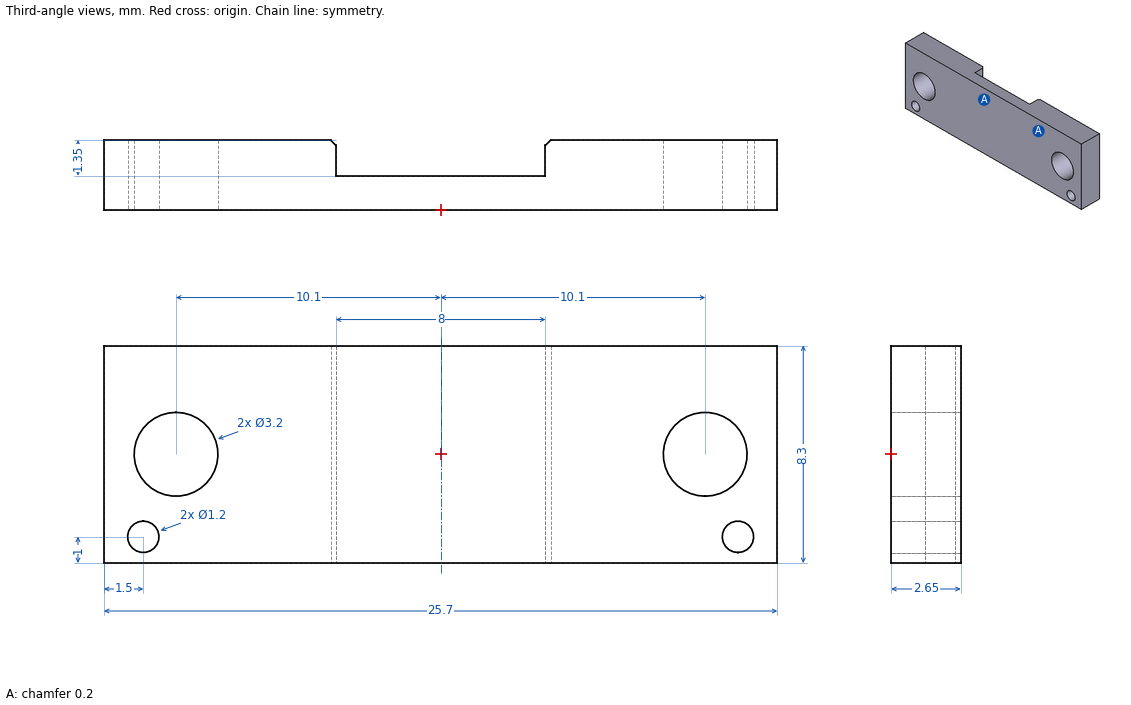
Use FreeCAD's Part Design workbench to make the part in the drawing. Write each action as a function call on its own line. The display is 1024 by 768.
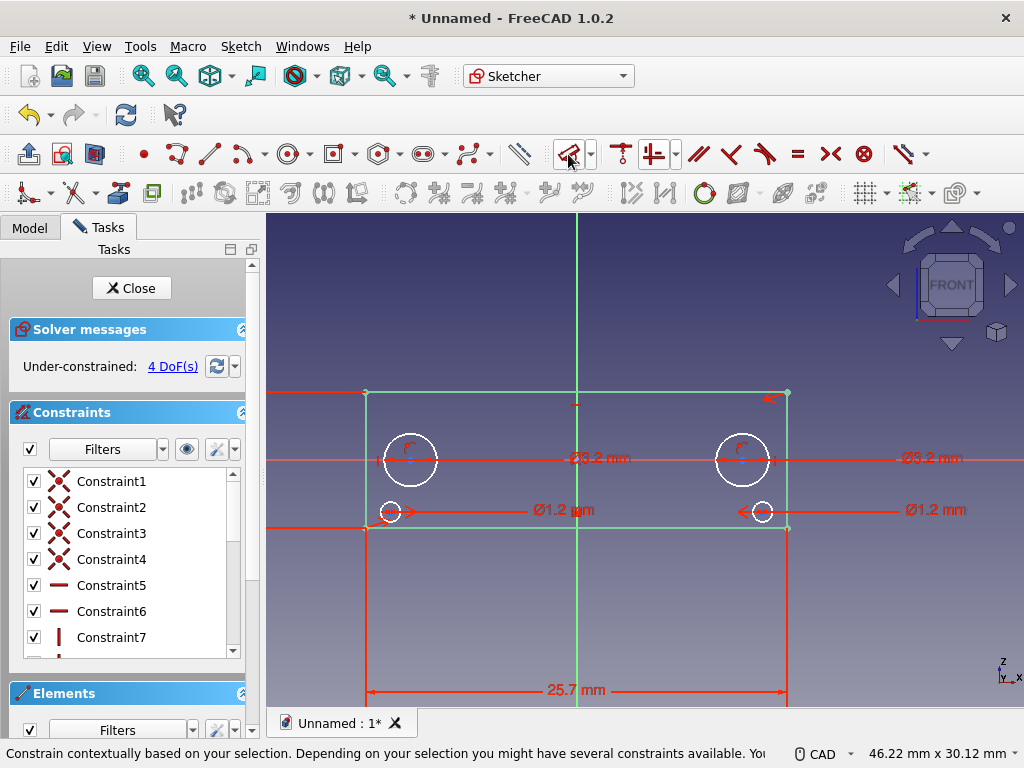
scroll(366, 528, up, 5)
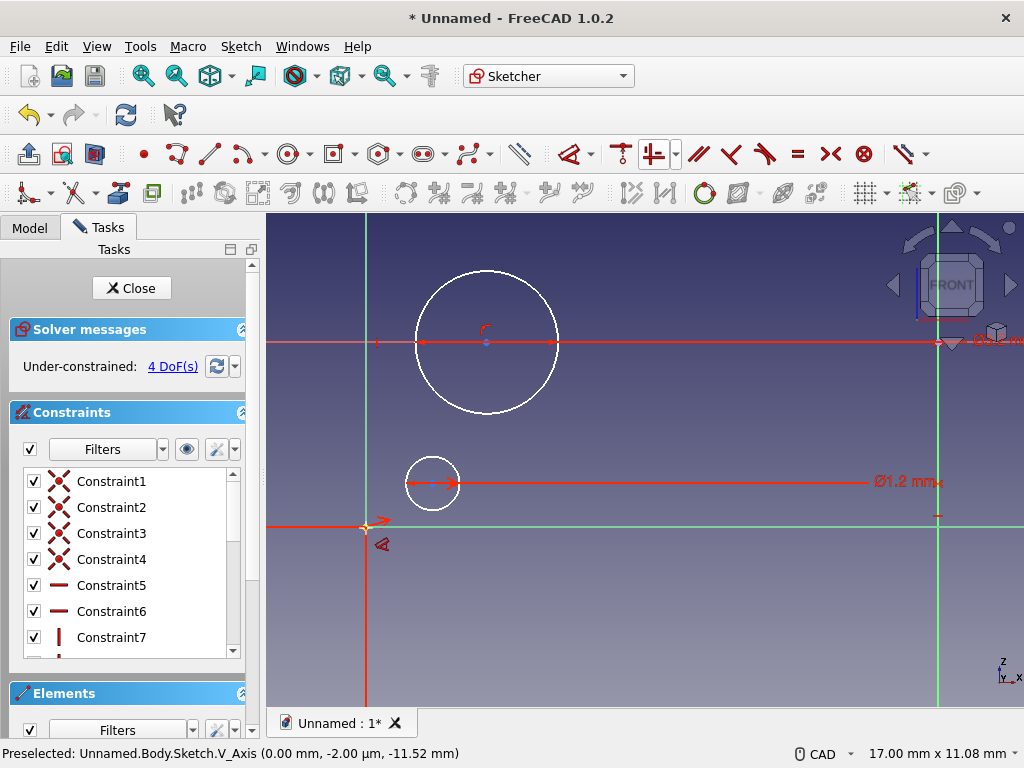
click(366, 527)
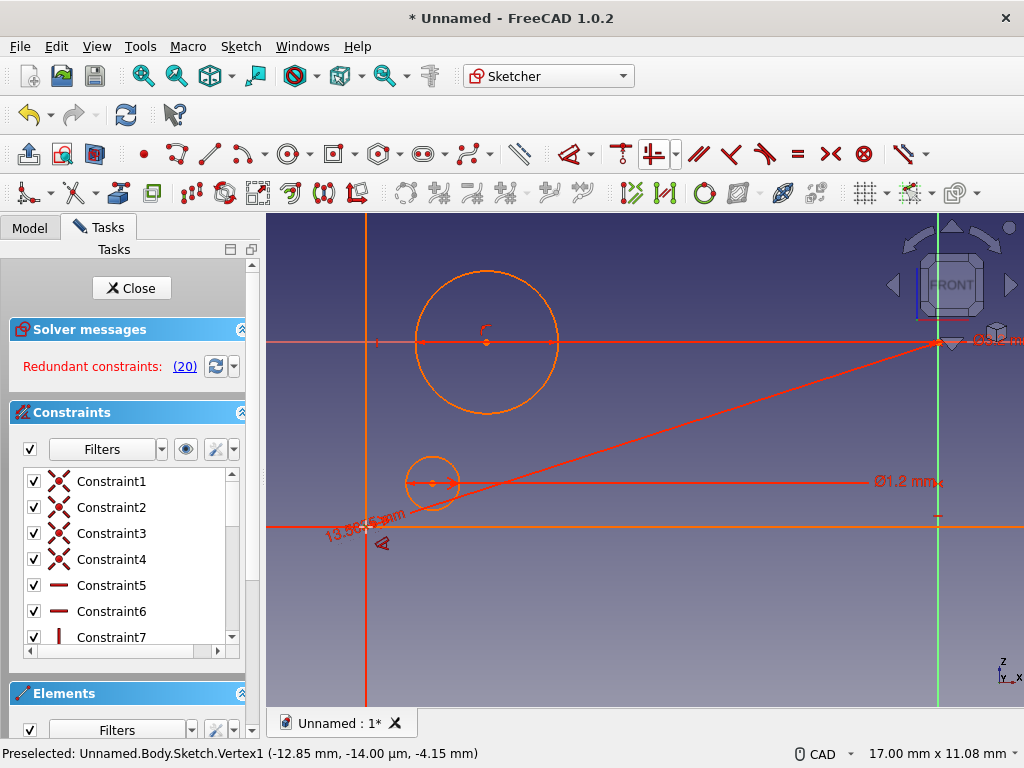
click(433, 483)
click(332, 505)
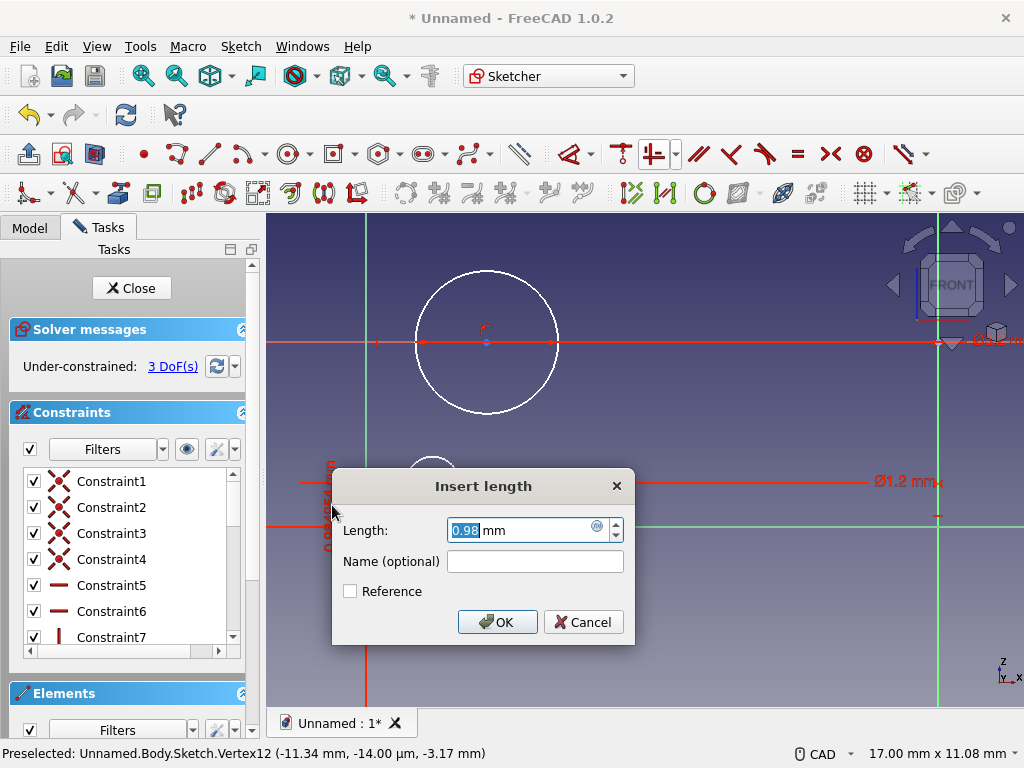
text(1)
key(Return)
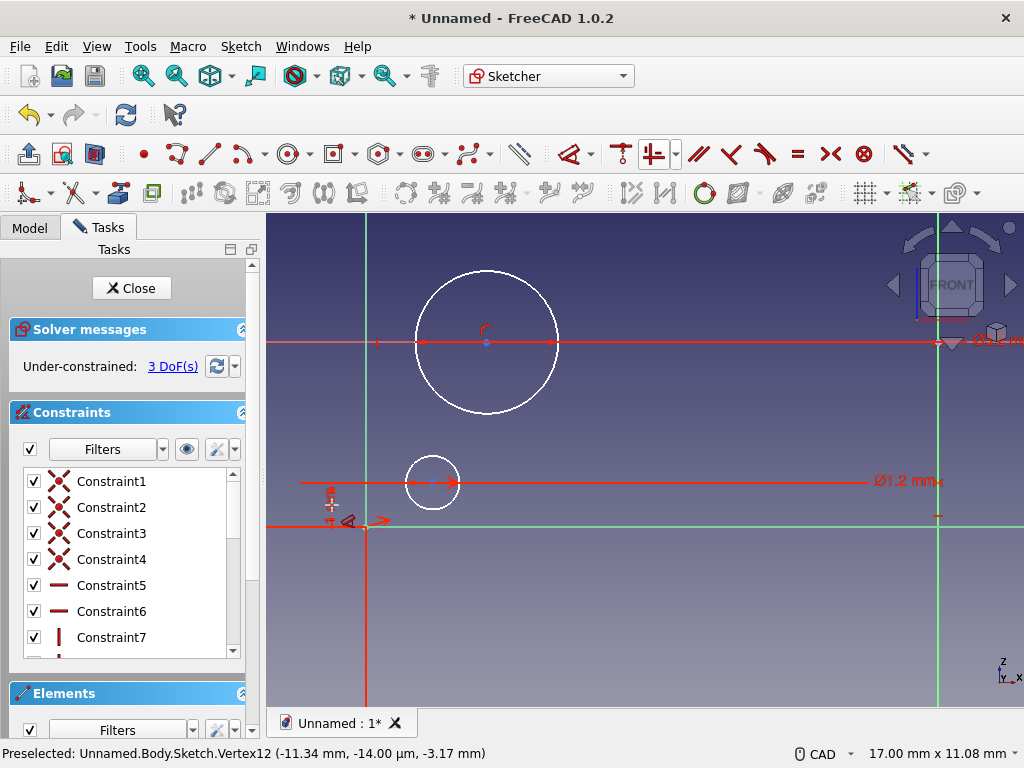
click(487, 342)
click(673, 376)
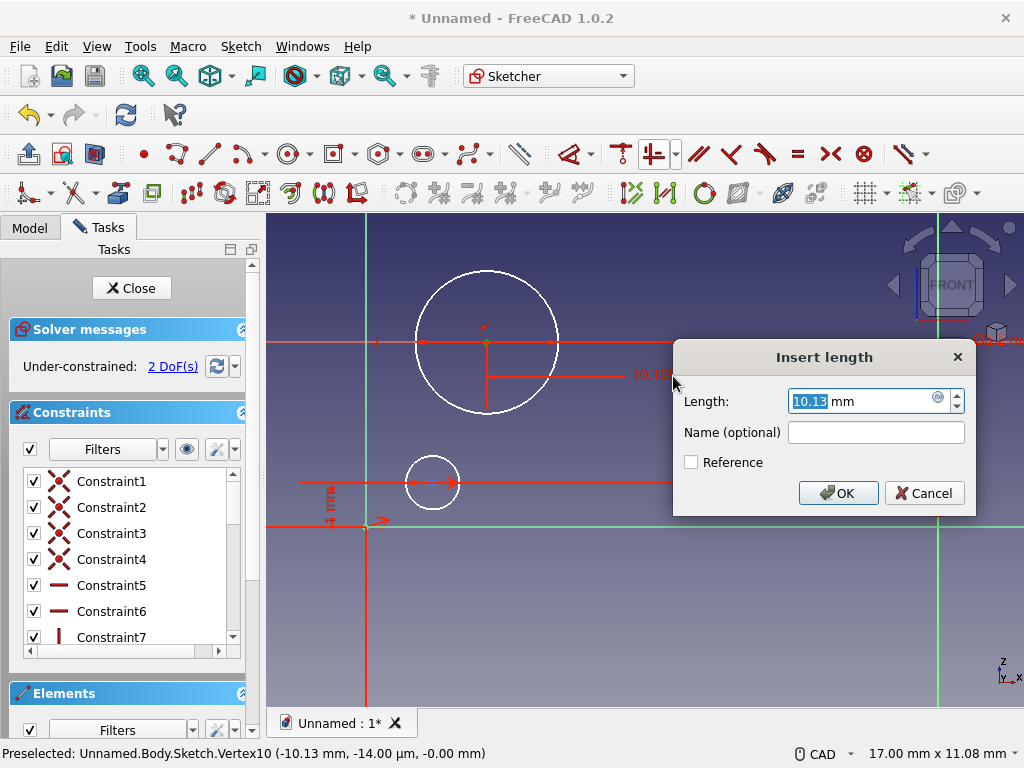
text(10.1)
key(Return)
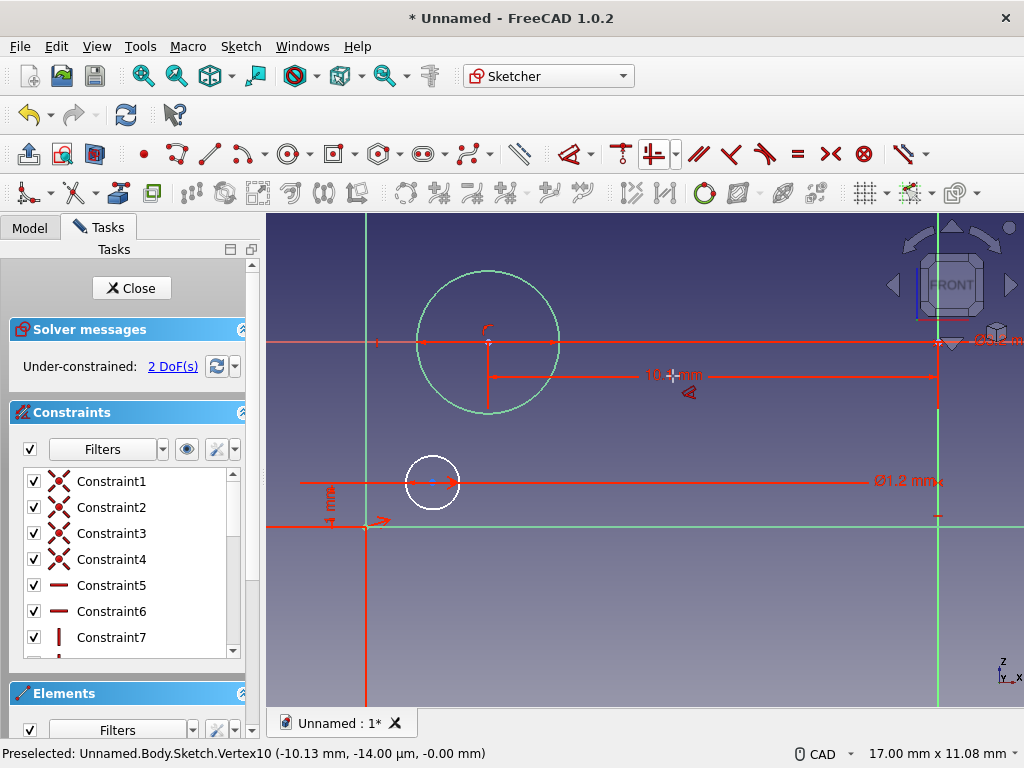
scroll(366, 528, down, 5)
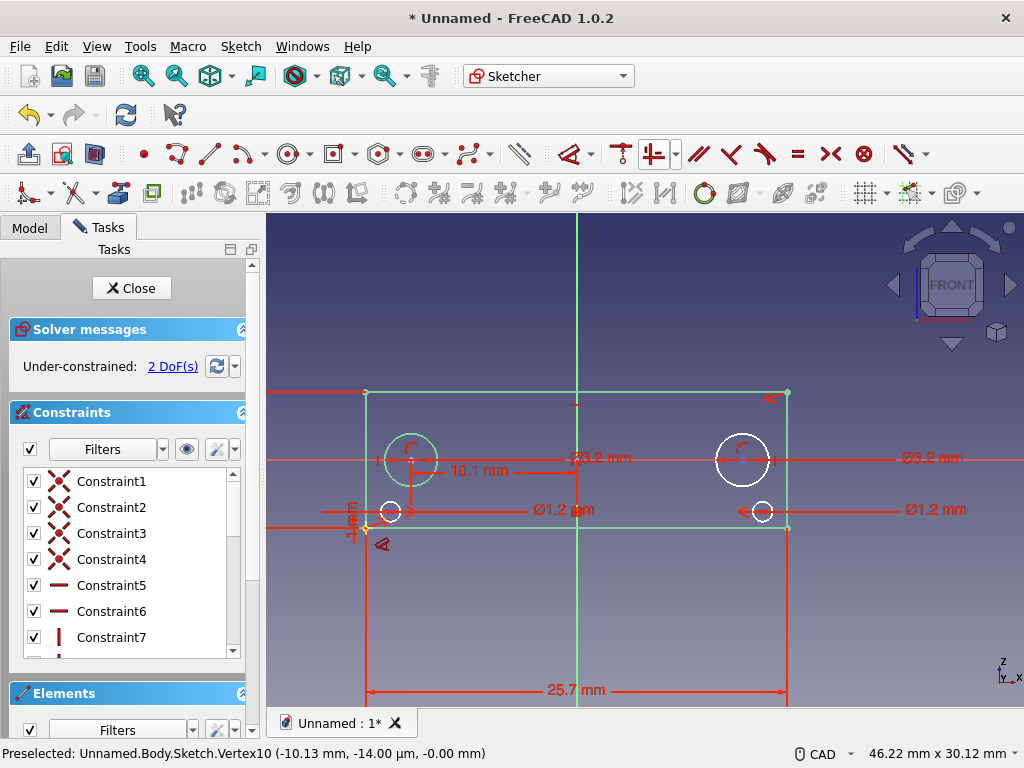
click(743, 460)
click(660, 494)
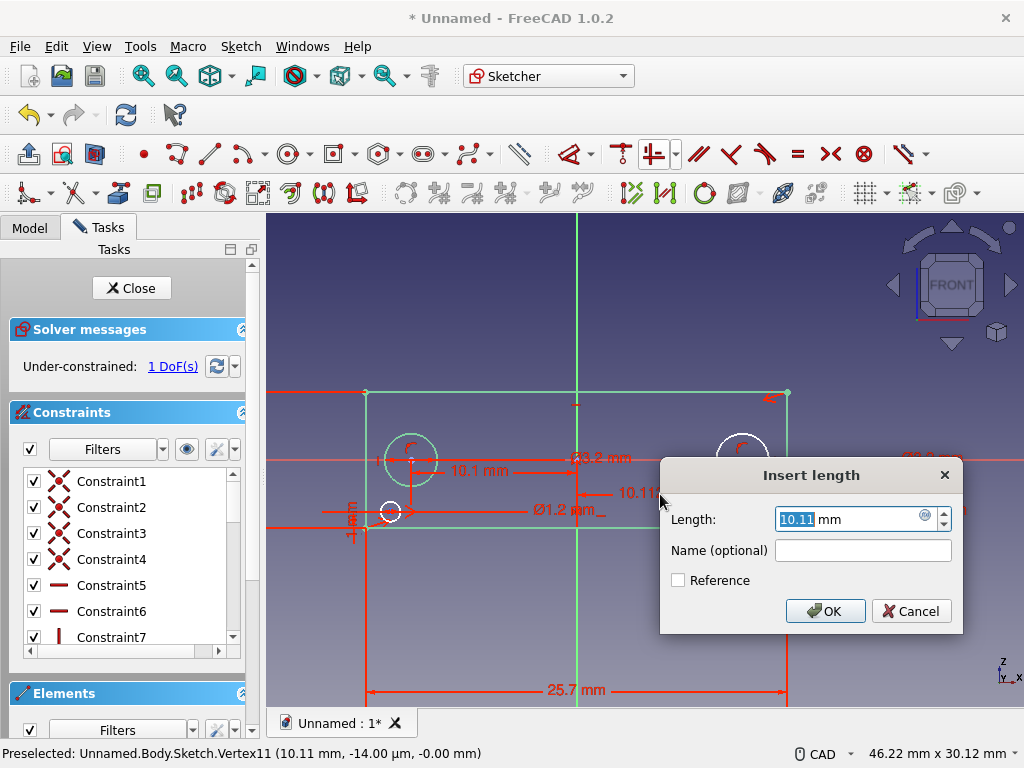
text(10.1)
key(Return)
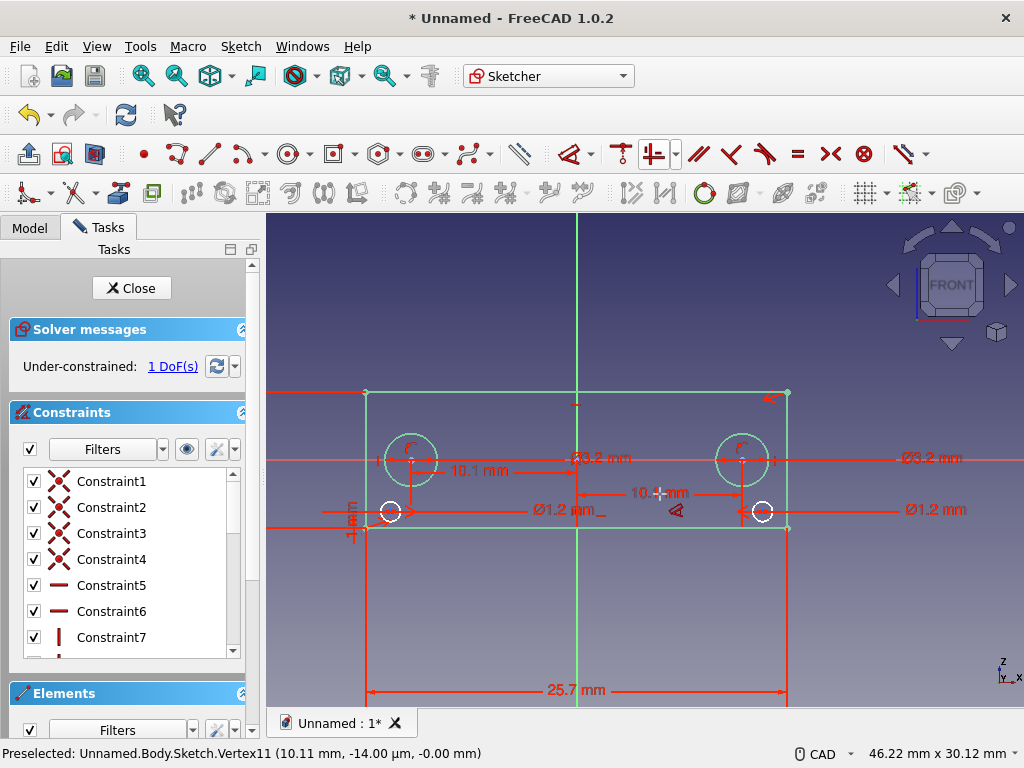
scroll(366, 528, up, 3)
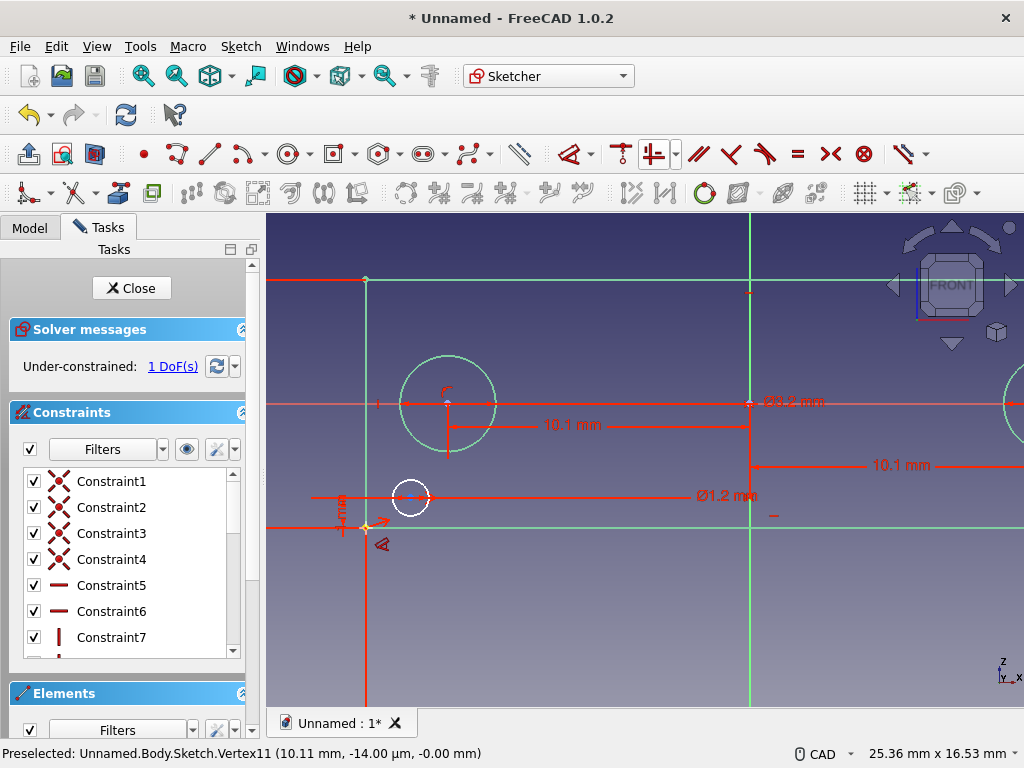
click(366, 528)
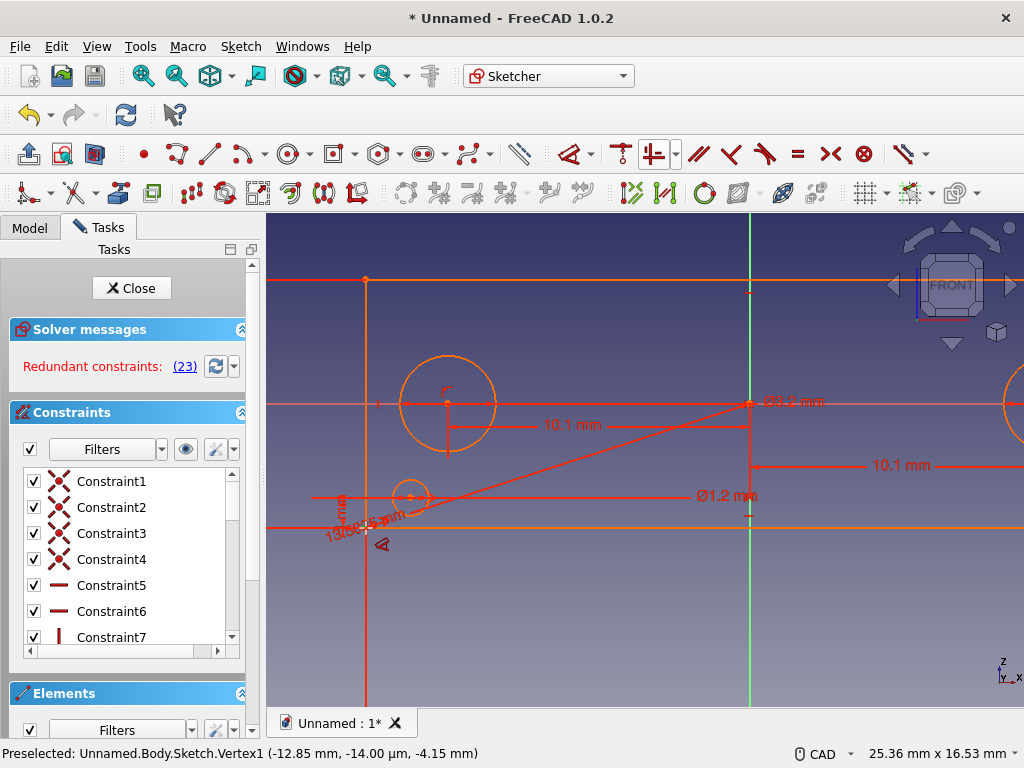
click(411, 498)
click(388, 562)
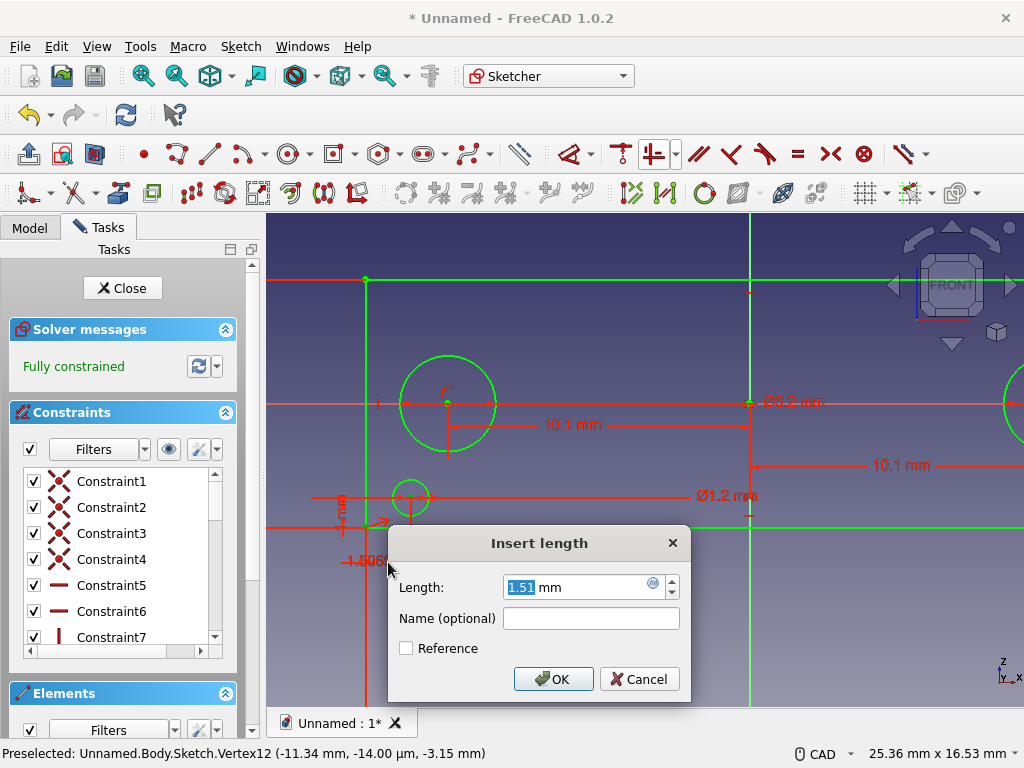
text(1.5)
key(Return)
key(Escape)